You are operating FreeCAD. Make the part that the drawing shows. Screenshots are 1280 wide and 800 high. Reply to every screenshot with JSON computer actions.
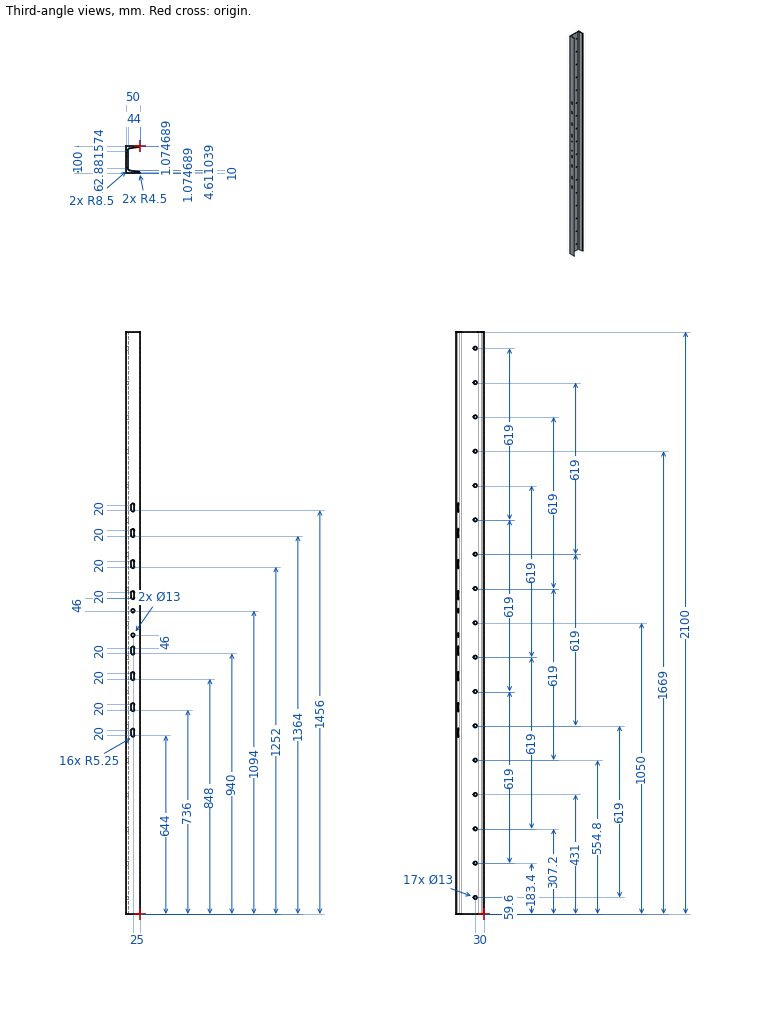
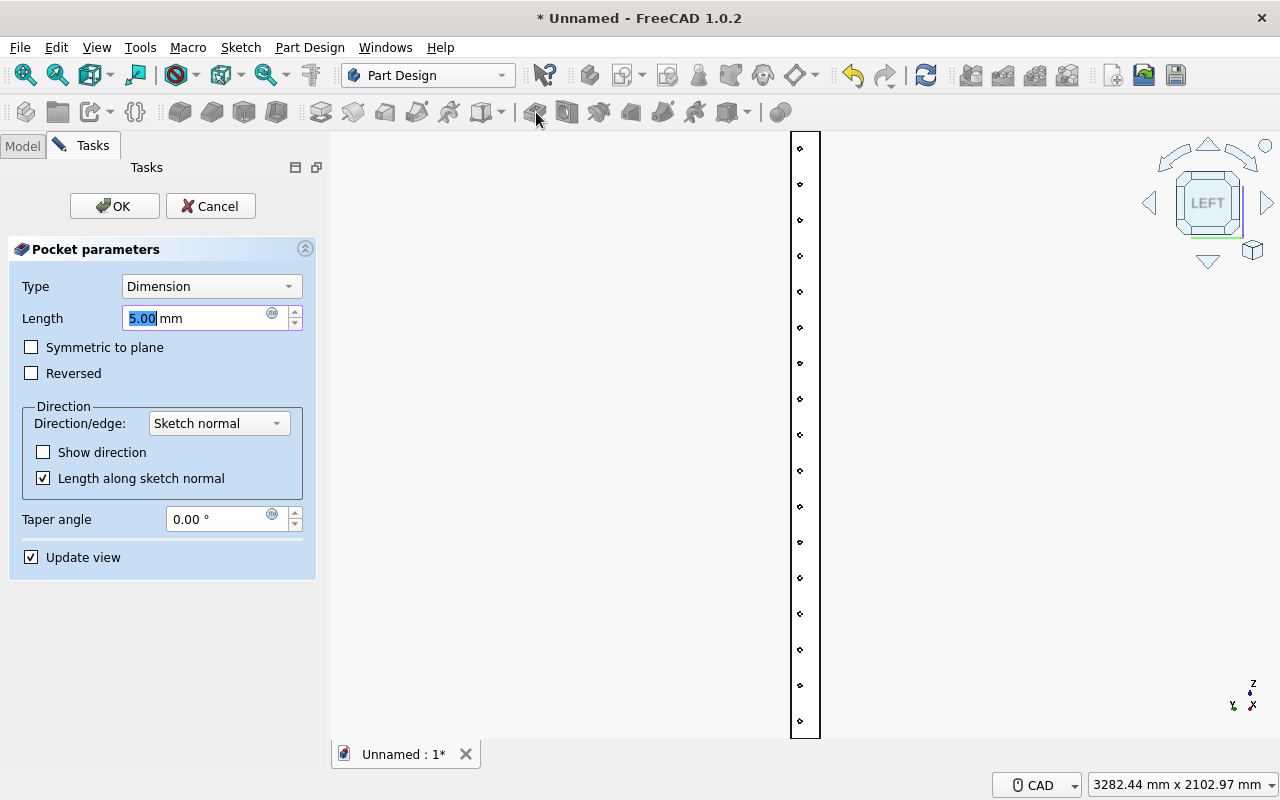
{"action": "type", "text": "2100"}
{"action": "key", "text": "Tab"}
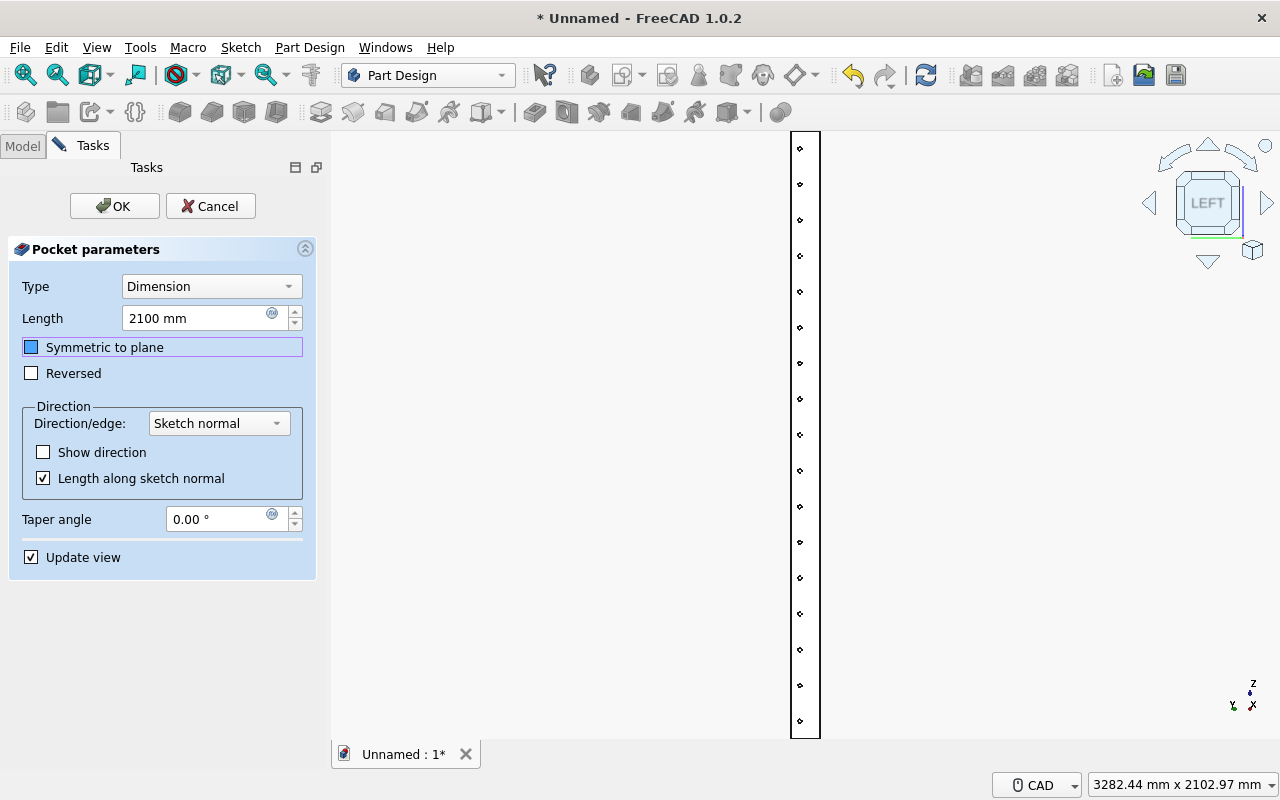
{"action": "left_click", "coordinate": [115, 206]}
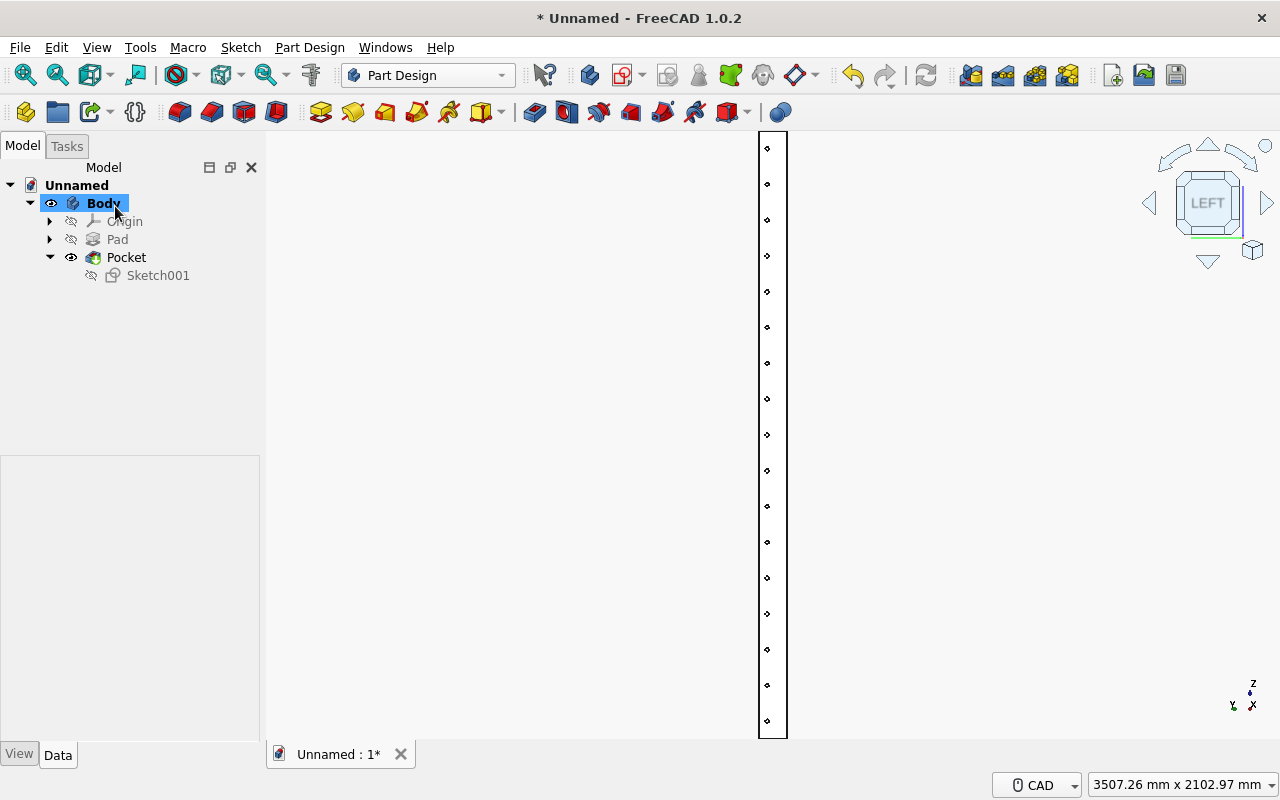
{"action": "left_click", "coordinate": [26, 76]}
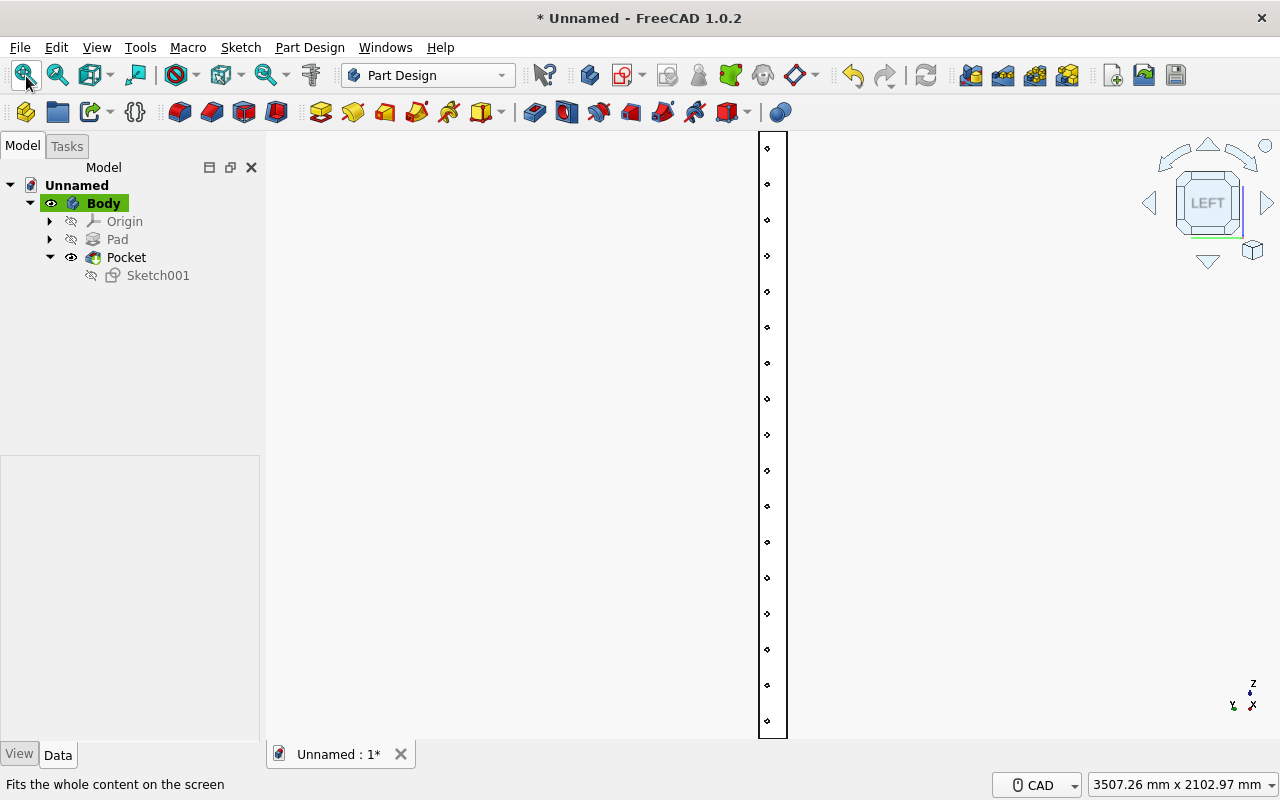
{"action": "key", "text": "0"}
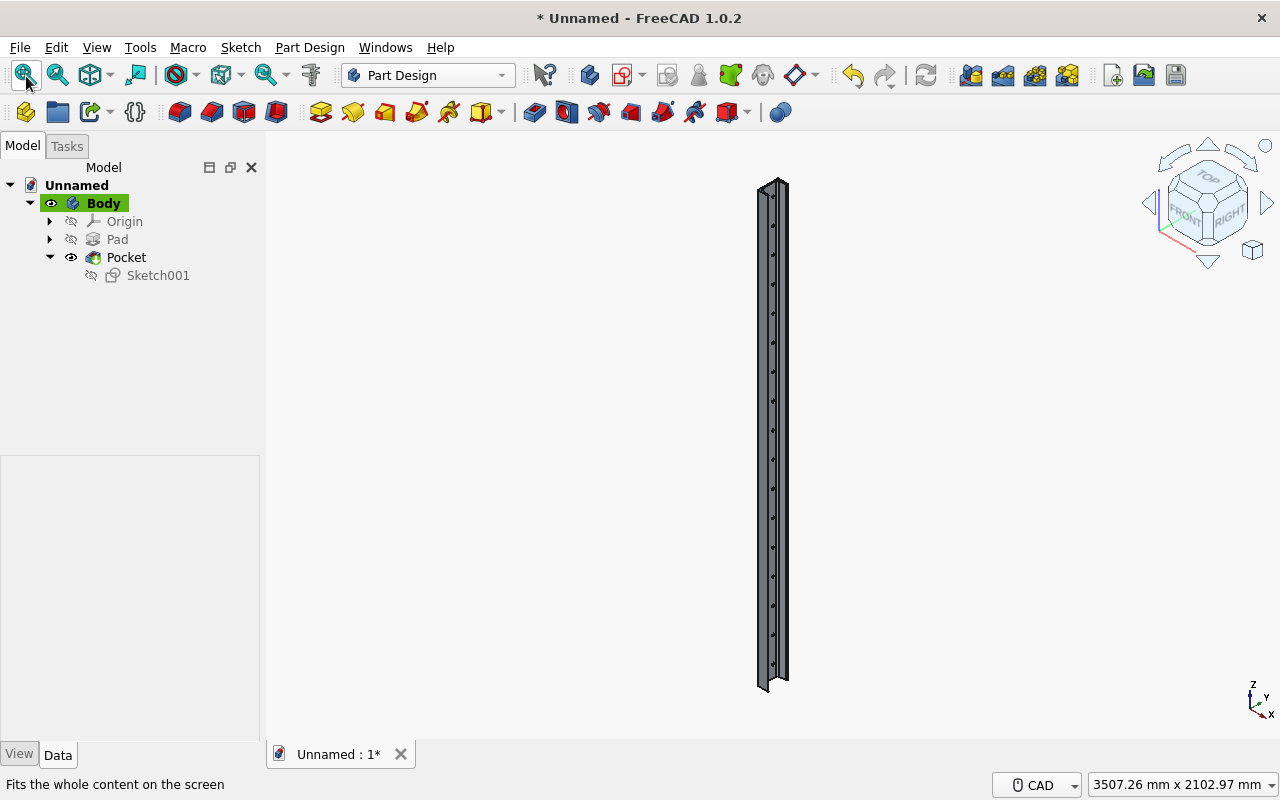
{"action": "key", "text": "1"}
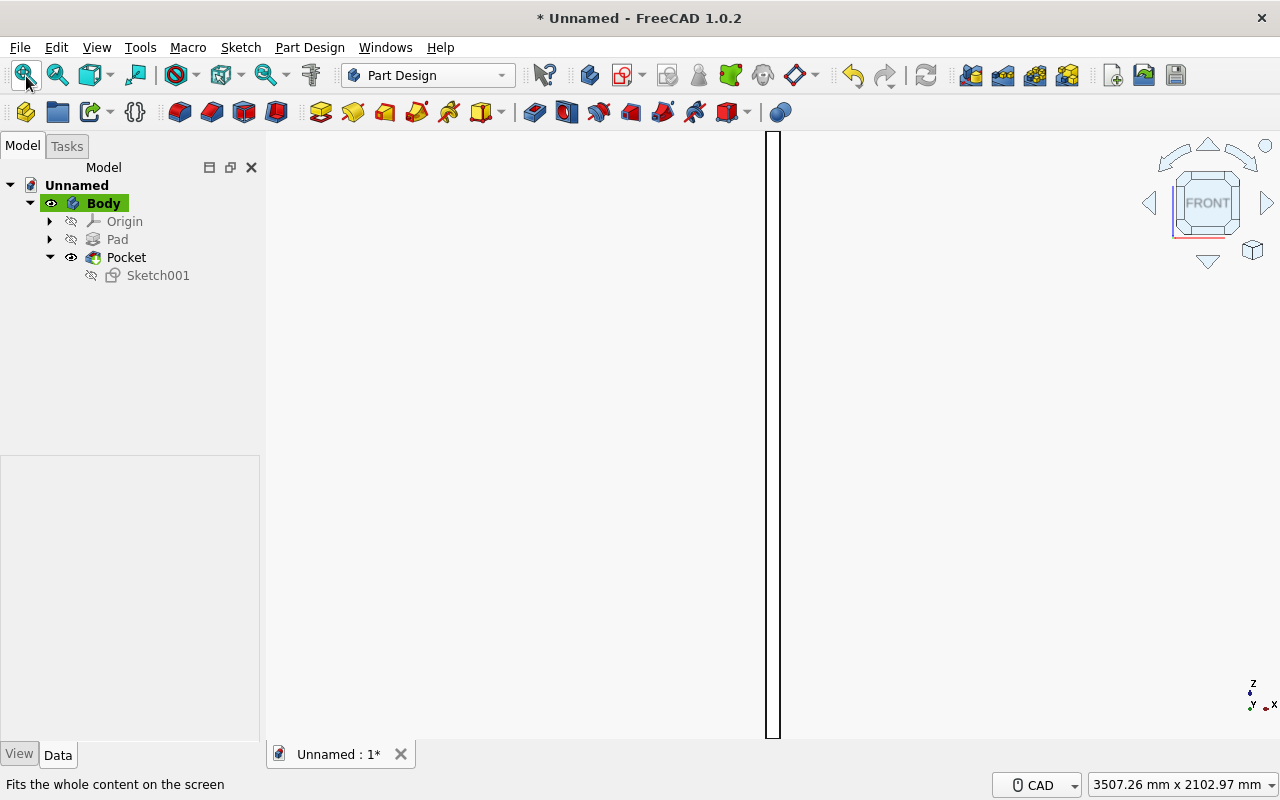
{"action": "left_click", "coordinate": [26, 76]}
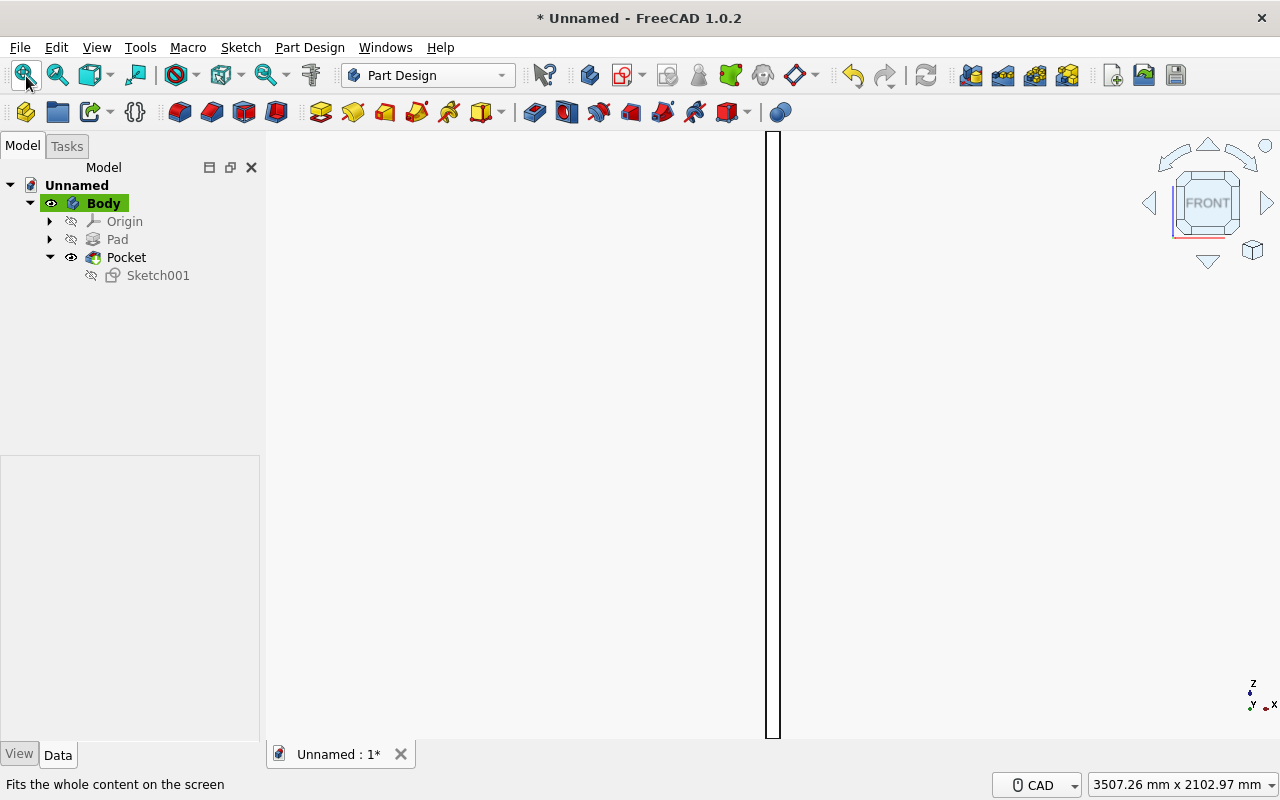
{"action": "key", "text": "2"}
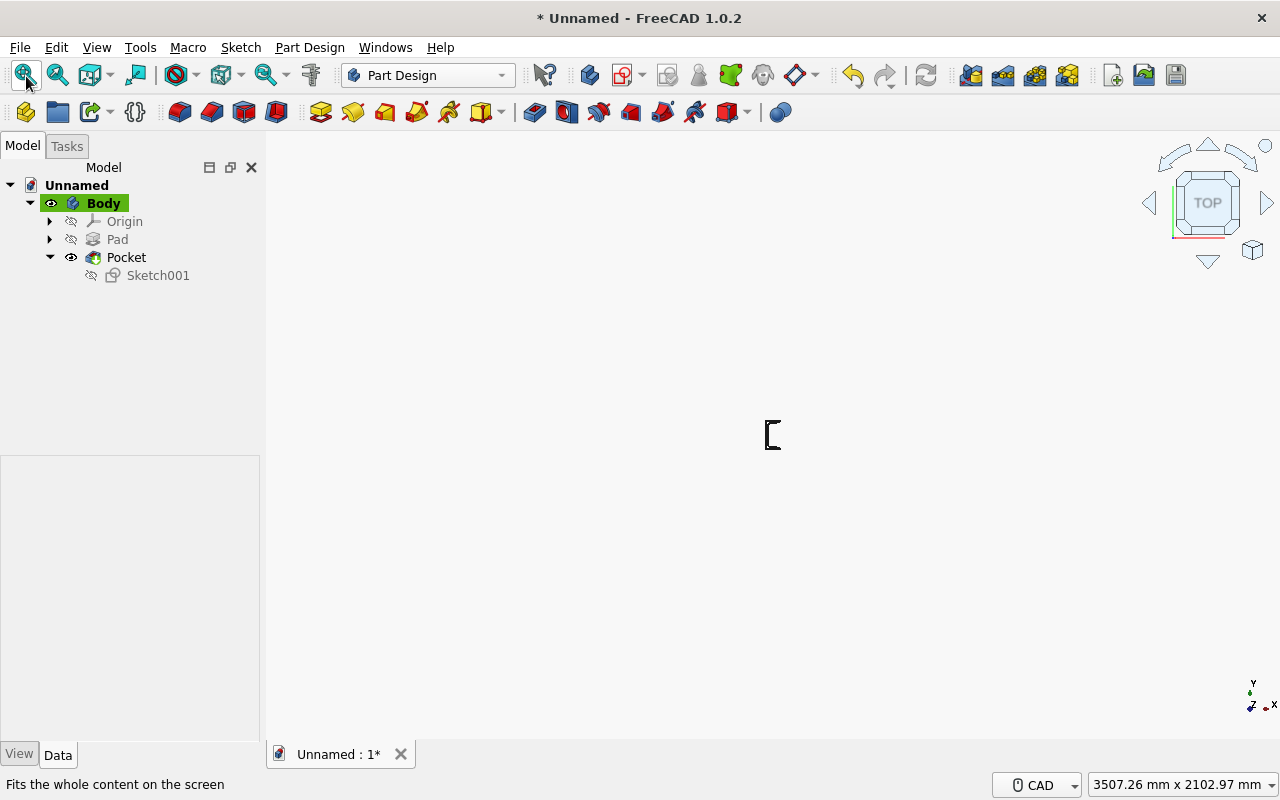
{"action": "left_click", "coordinate": [26, 76]}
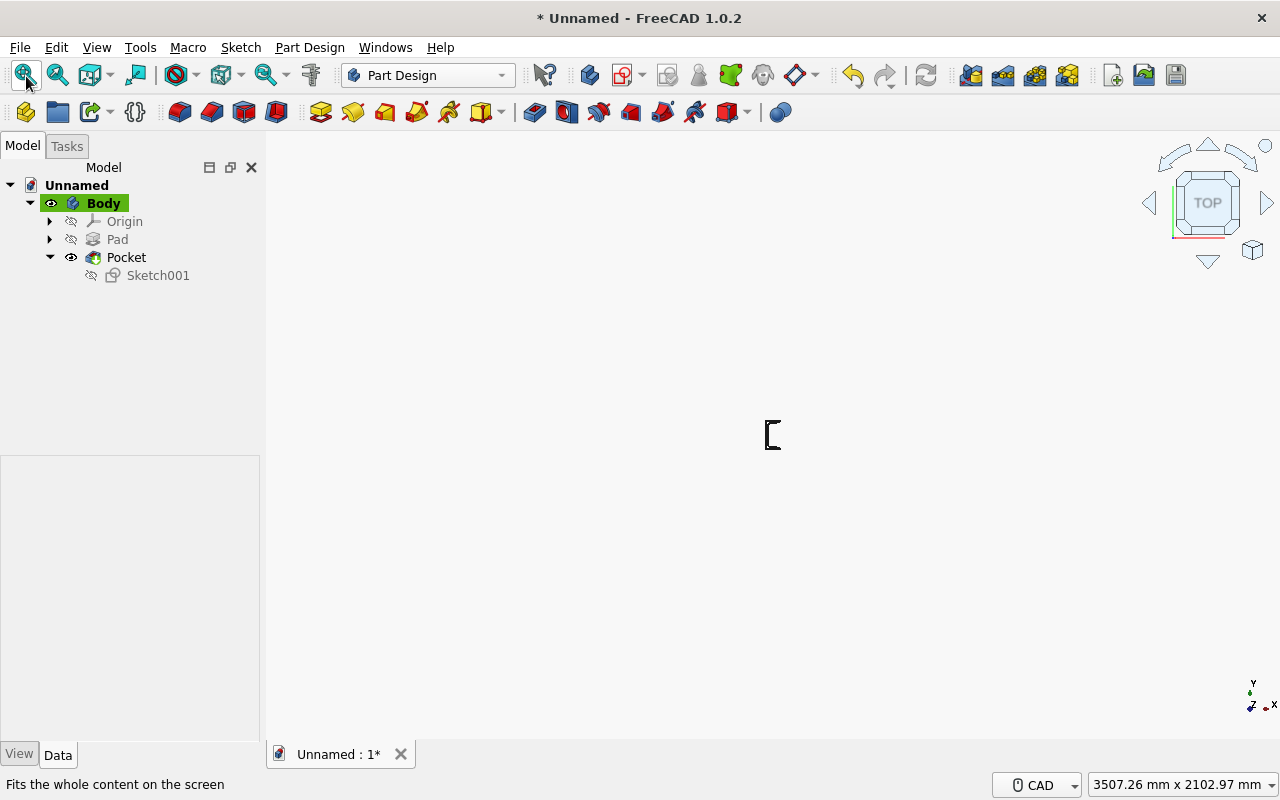
{"action": "left_click", "coordinate": [50, 221]}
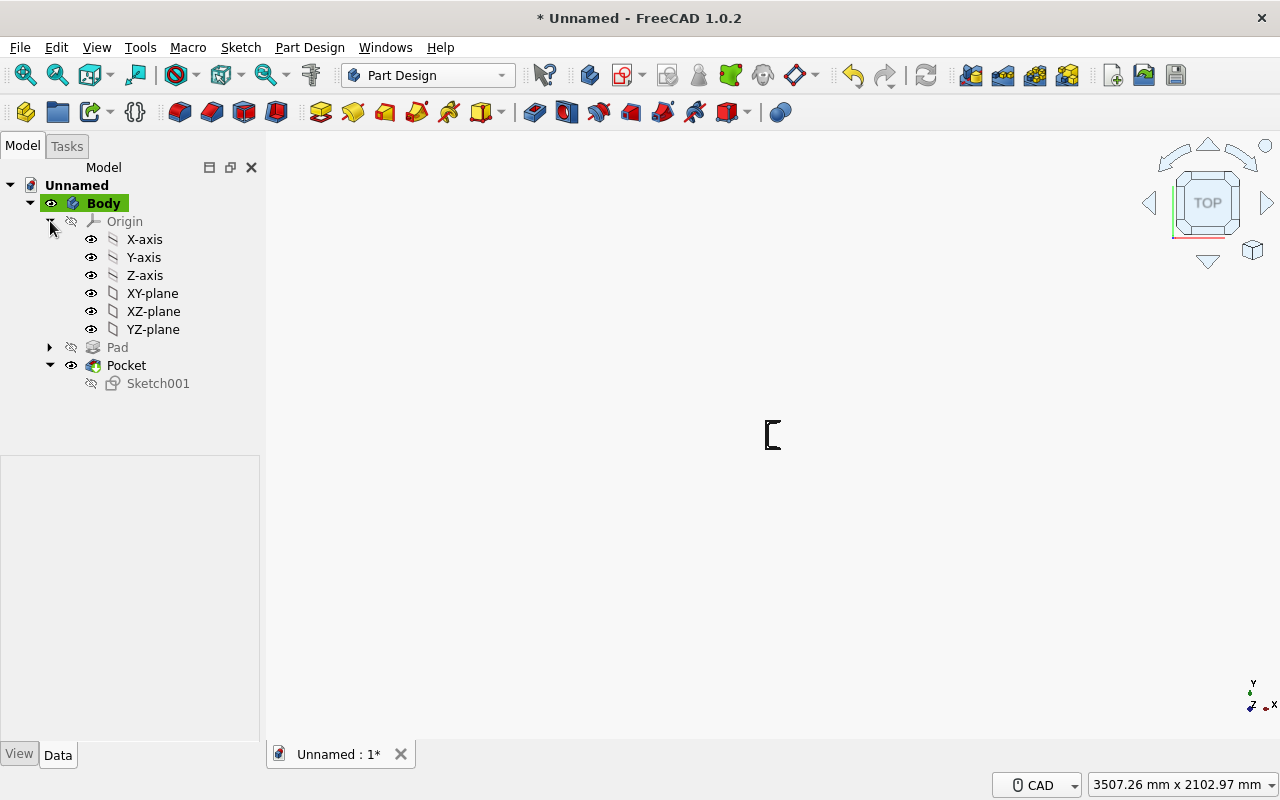
{"action": "left_click", "coordinate": [136, 311]}